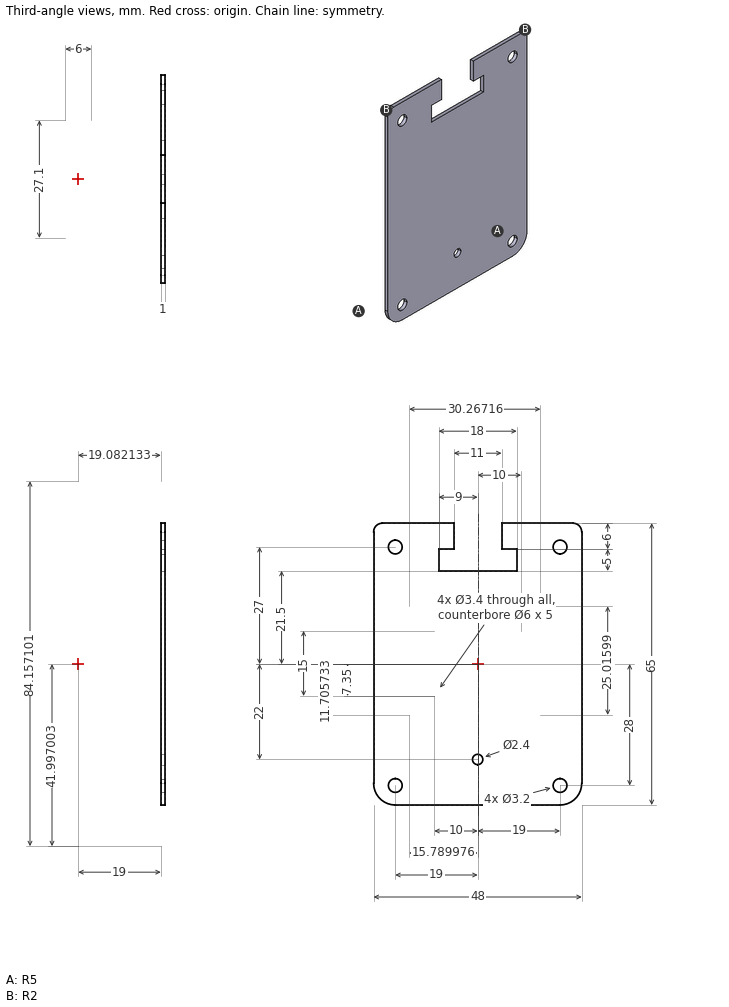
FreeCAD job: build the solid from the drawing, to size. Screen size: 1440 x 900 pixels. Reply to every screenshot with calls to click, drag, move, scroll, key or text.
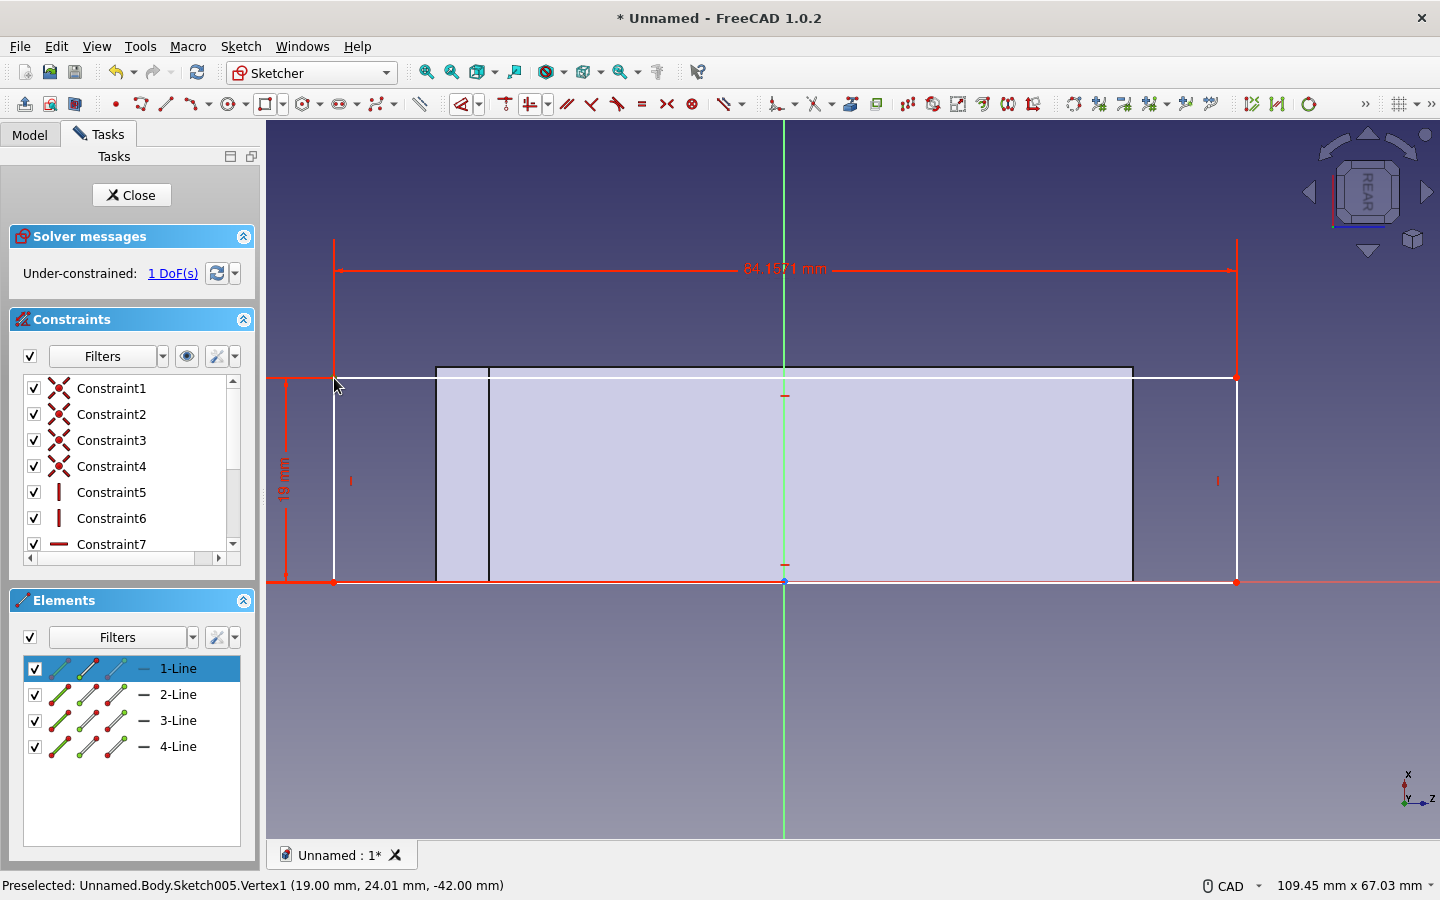
key(l)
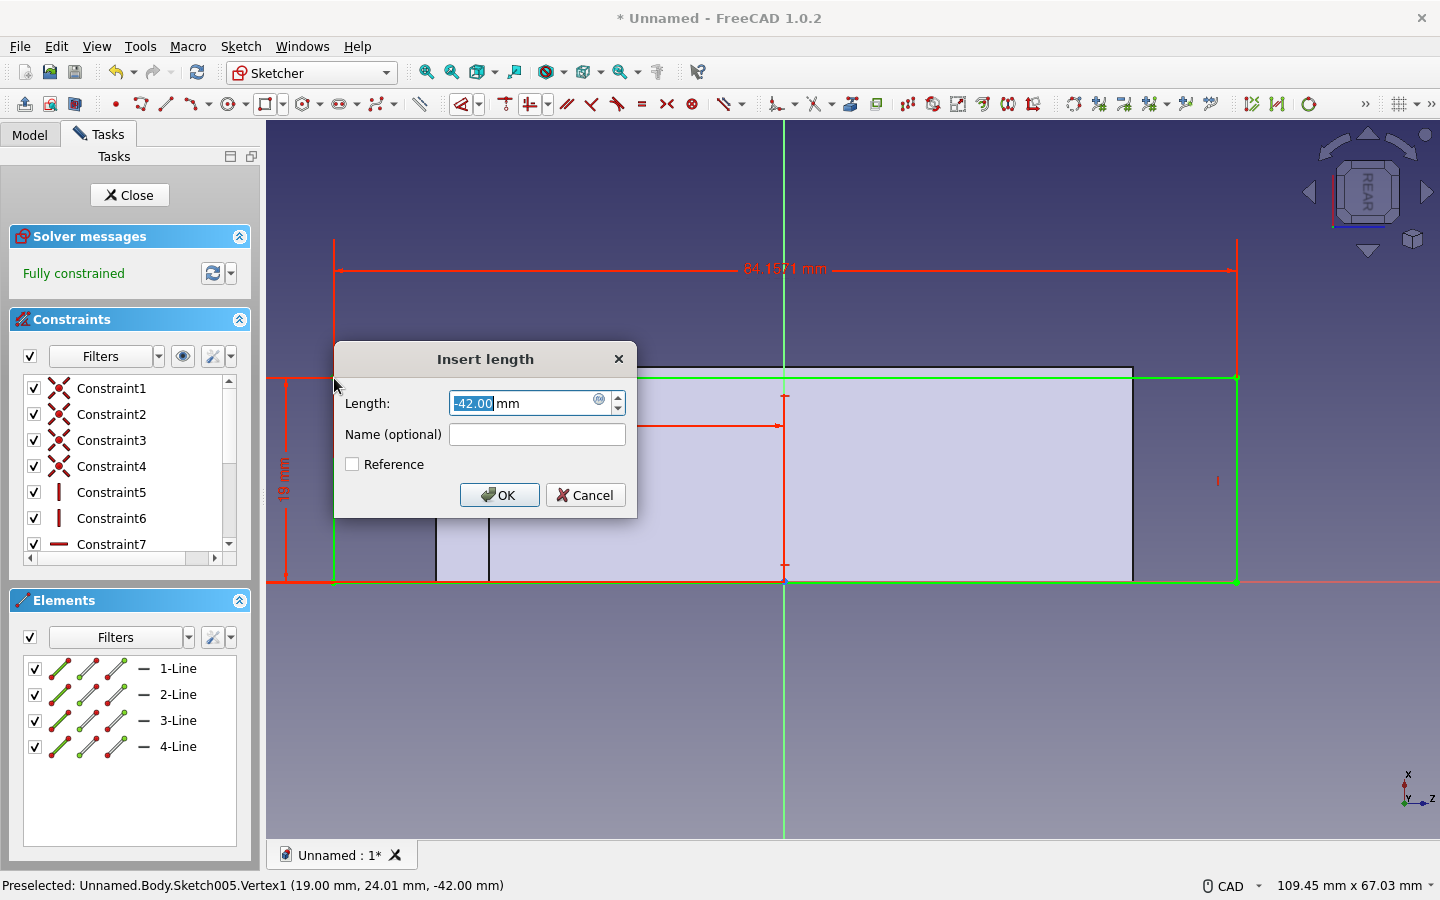
text(-41.997003)
key(Return)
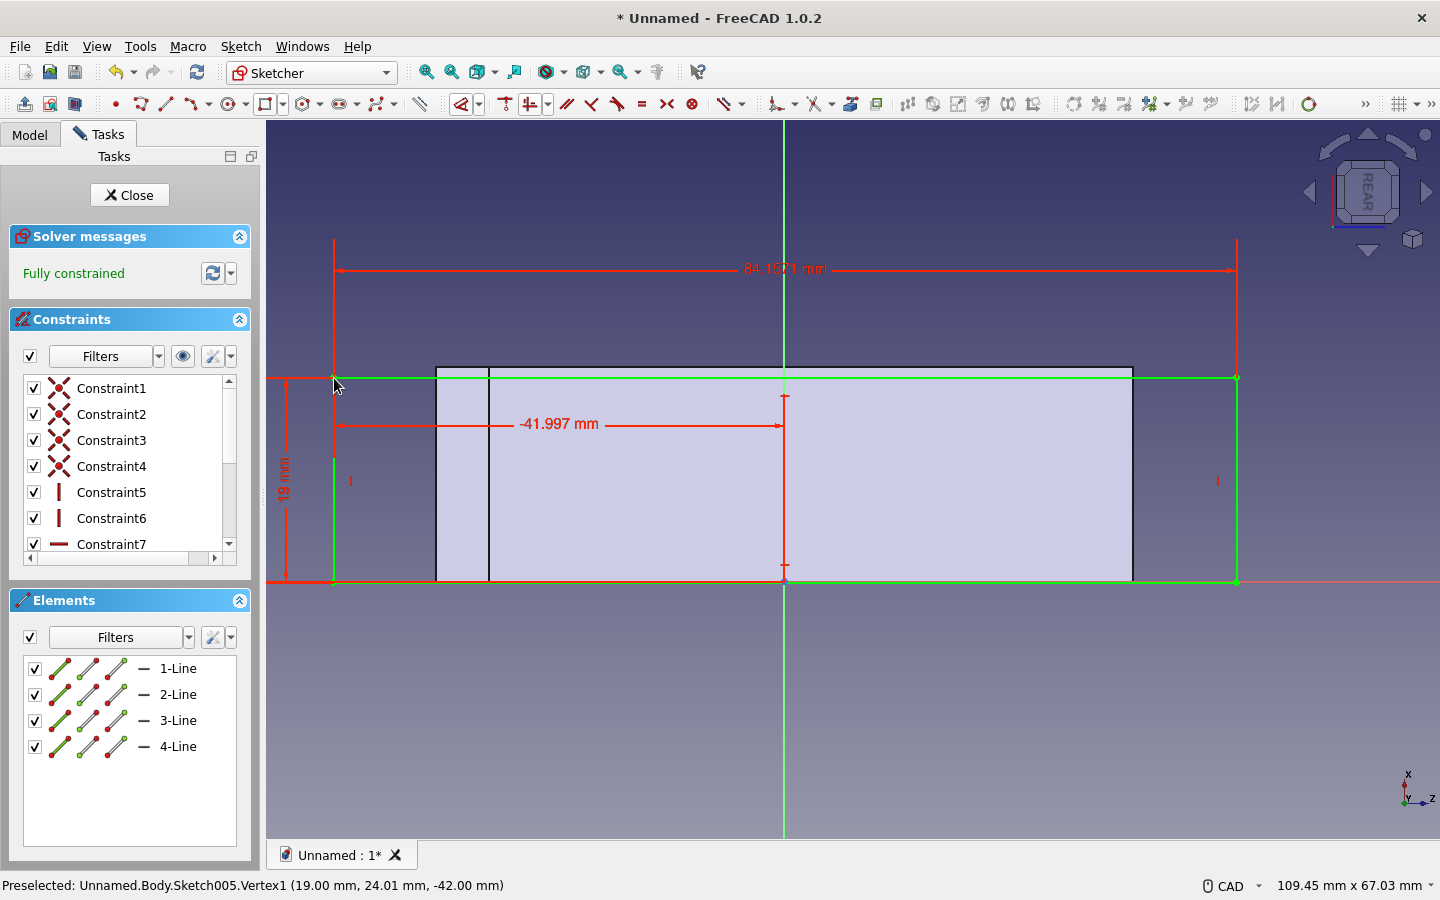
click(130, 195)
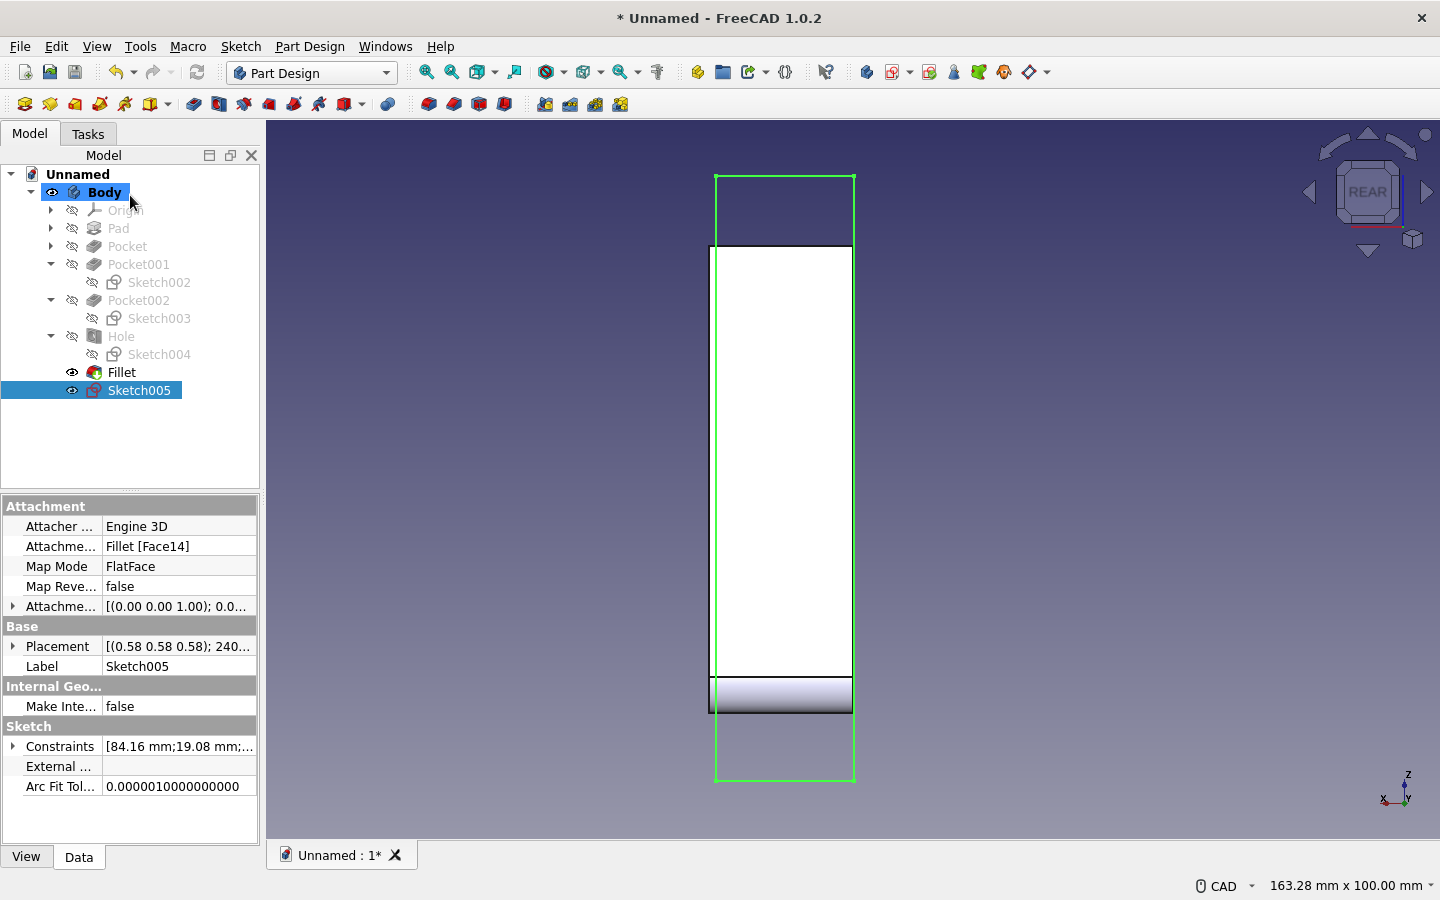
click(194, 104)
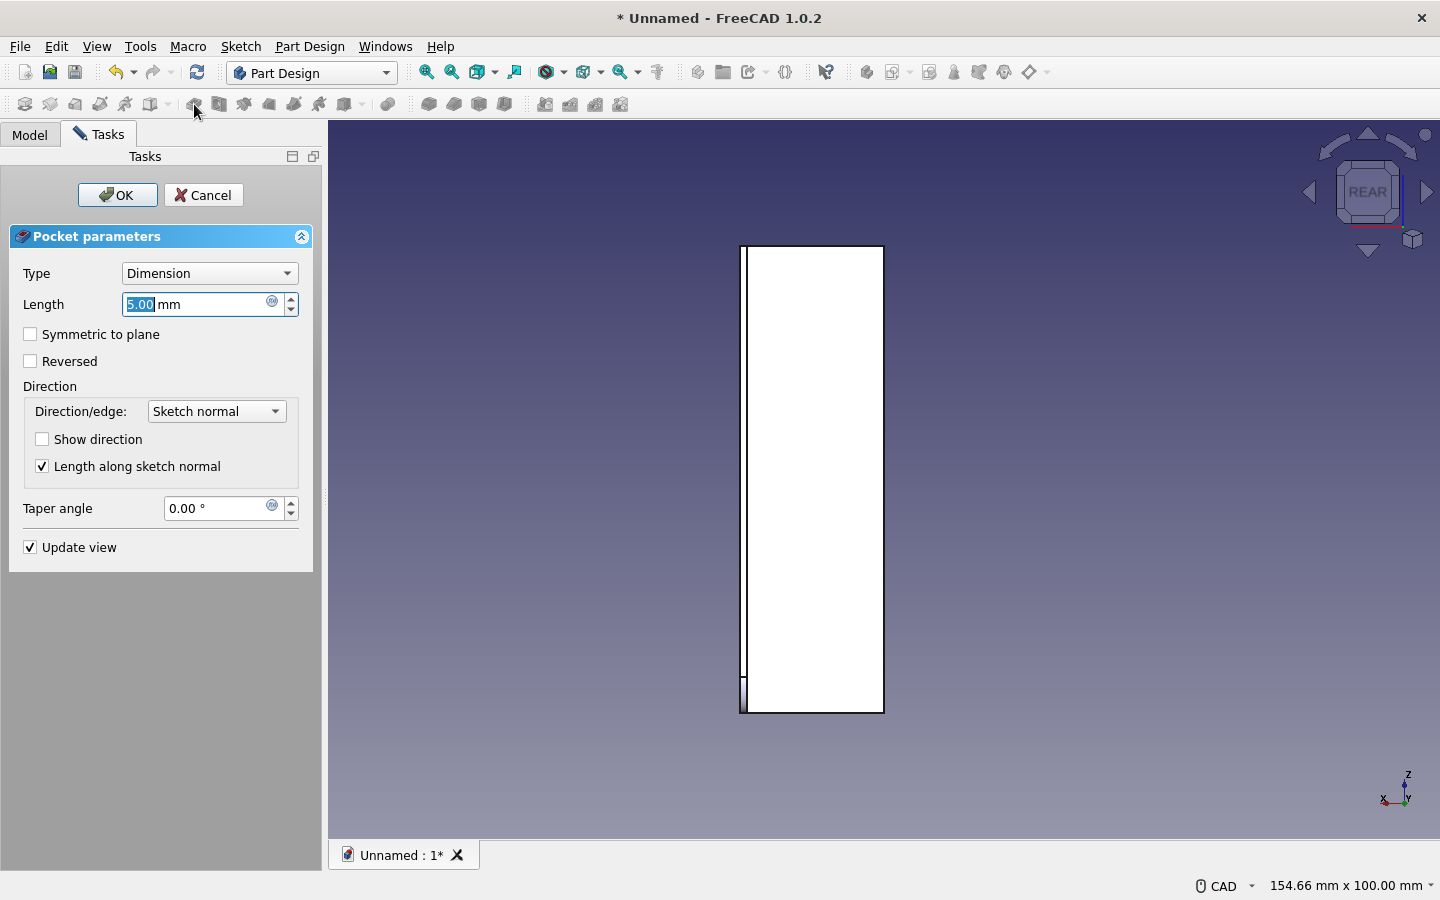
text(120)
key(Tab)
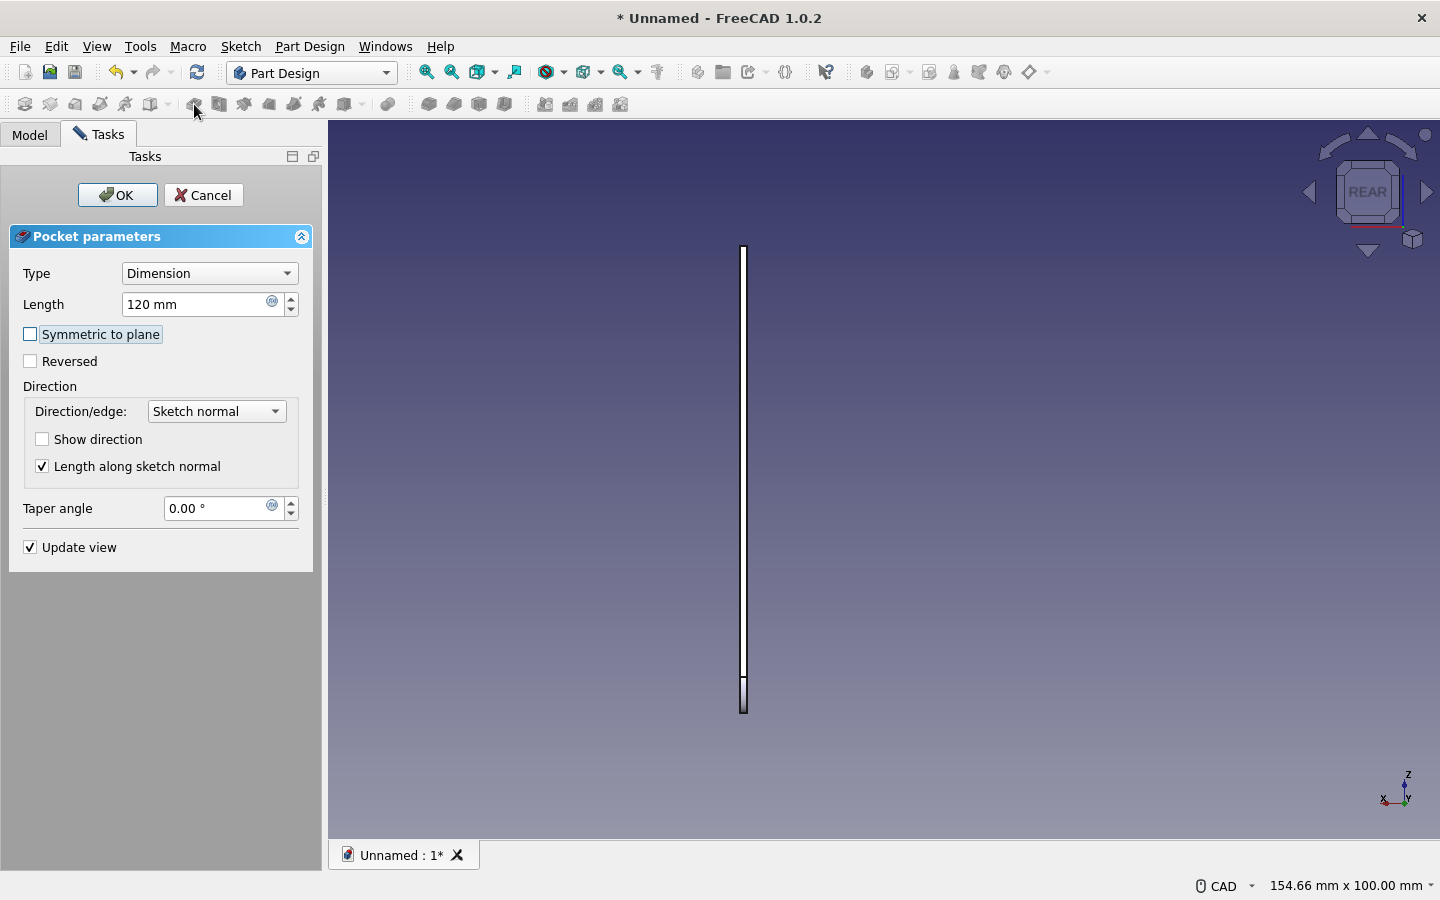
click(118, 195)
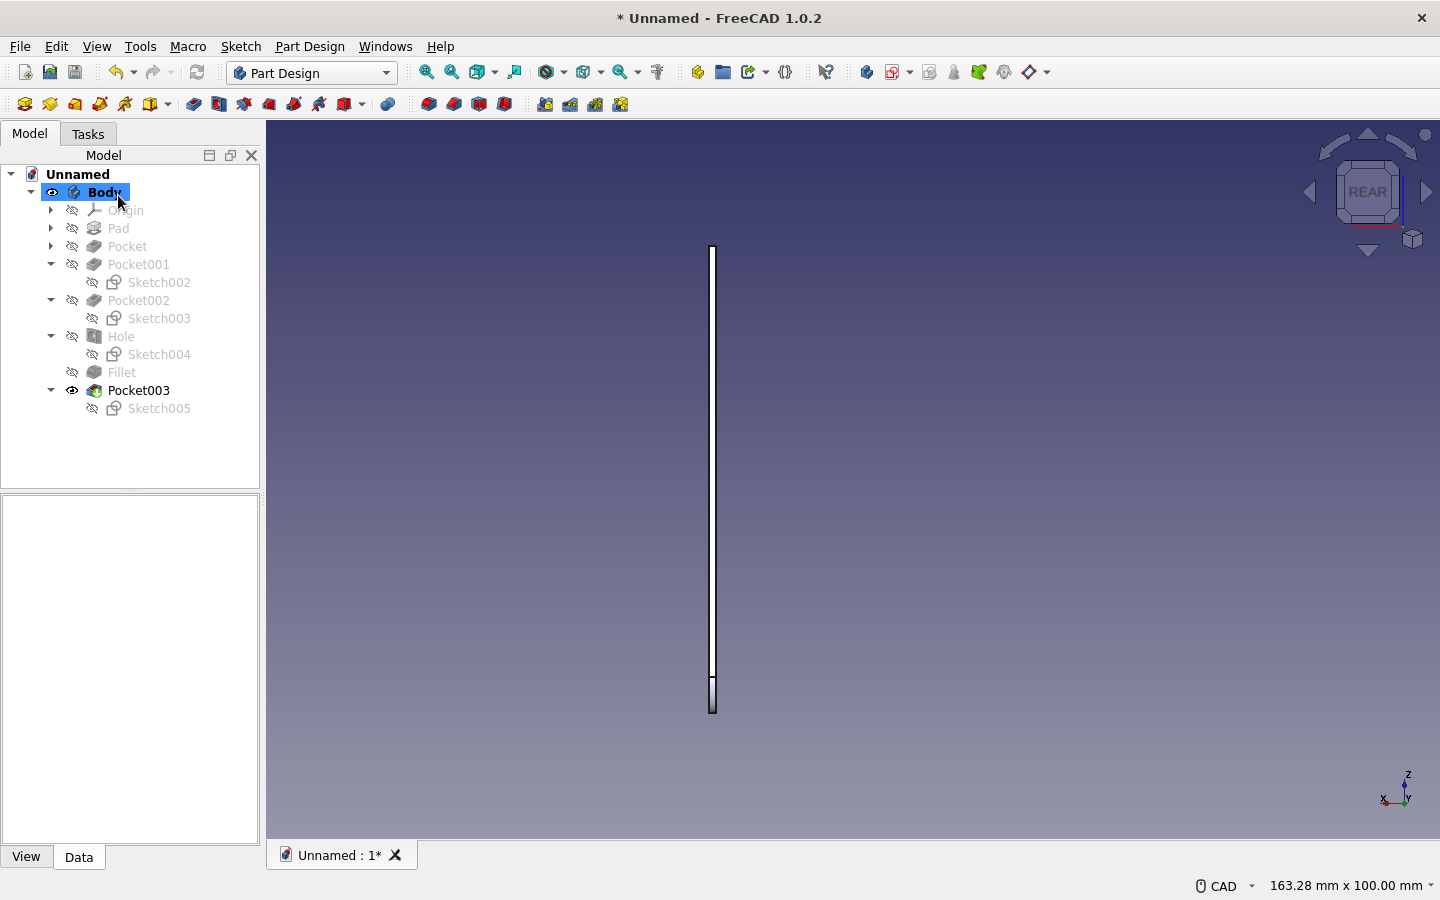
key(6)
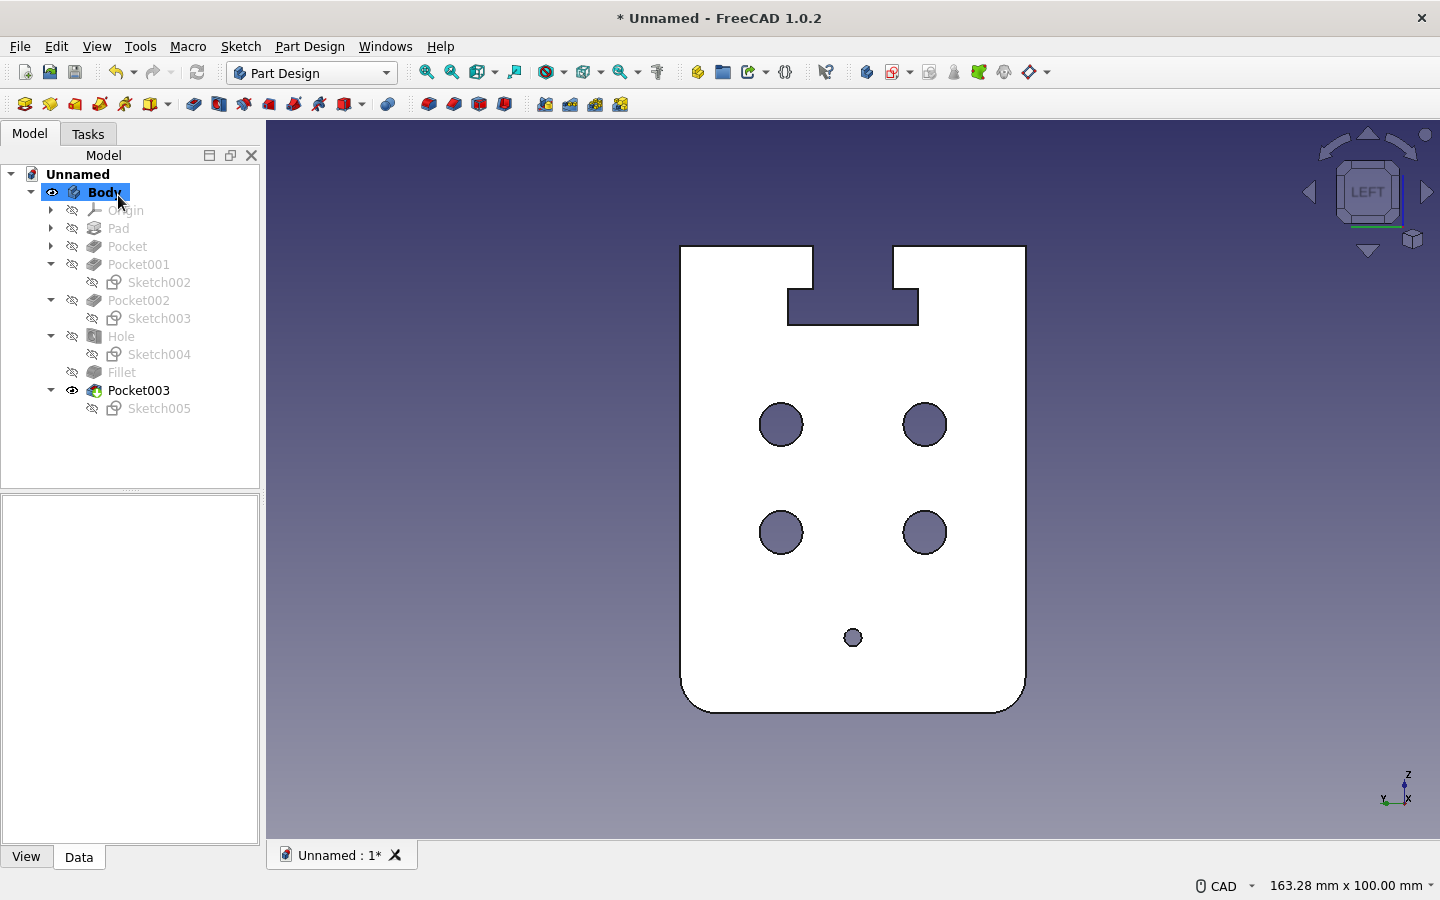
click(853, 479)